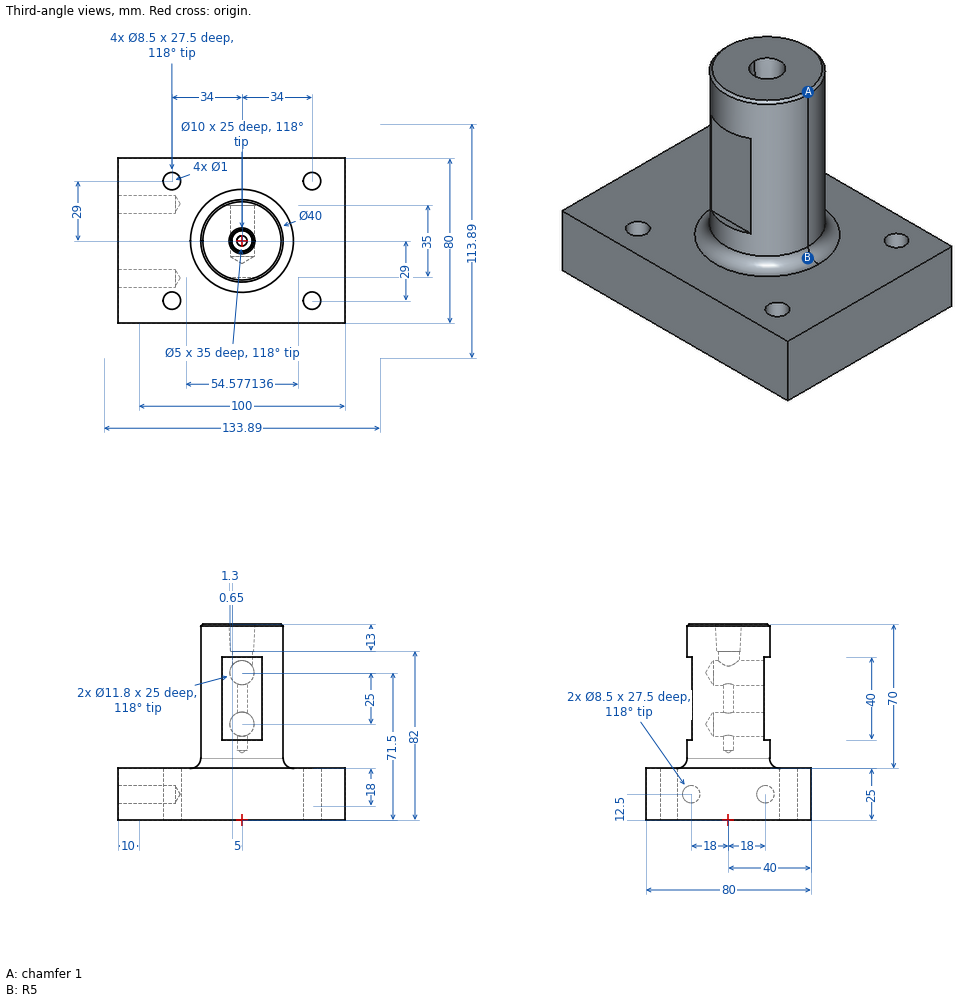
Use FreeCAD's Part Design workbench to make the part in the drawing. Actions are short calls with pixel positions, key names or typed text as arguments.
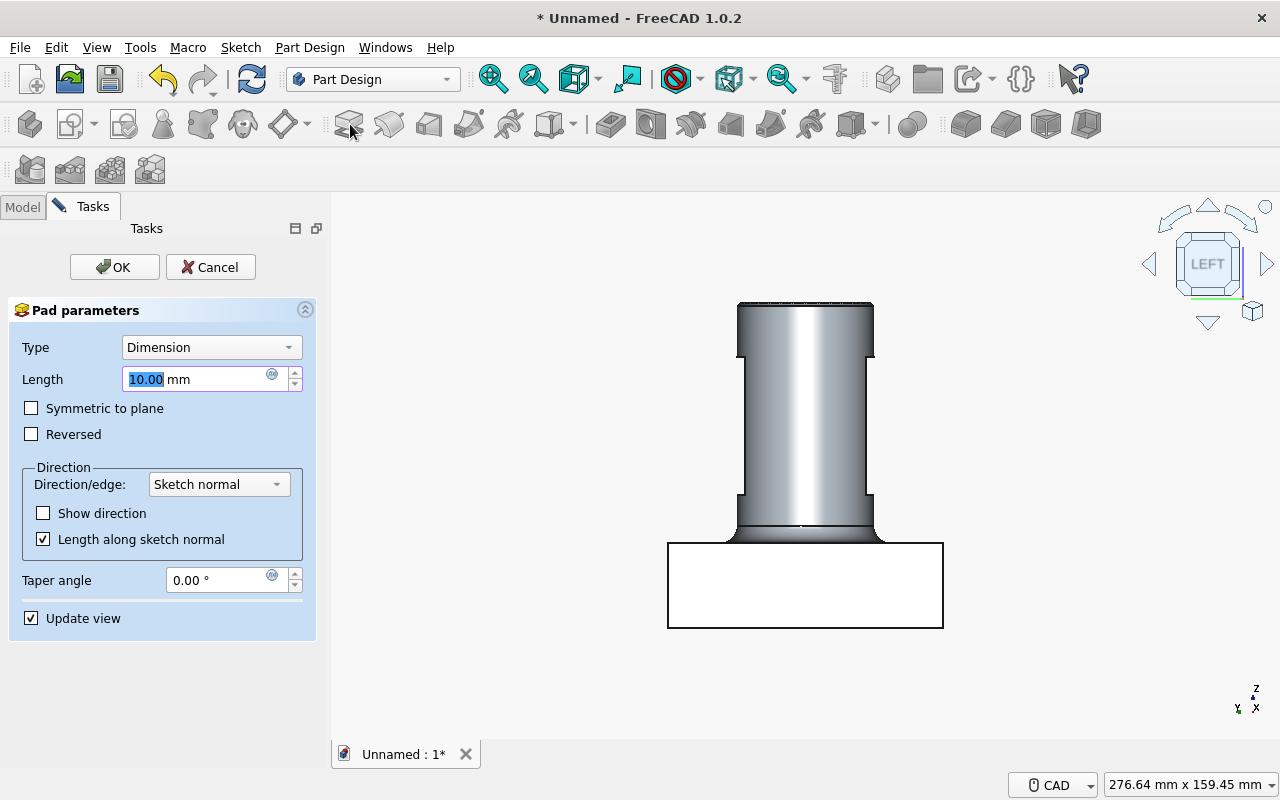
text(10)
key(Tab)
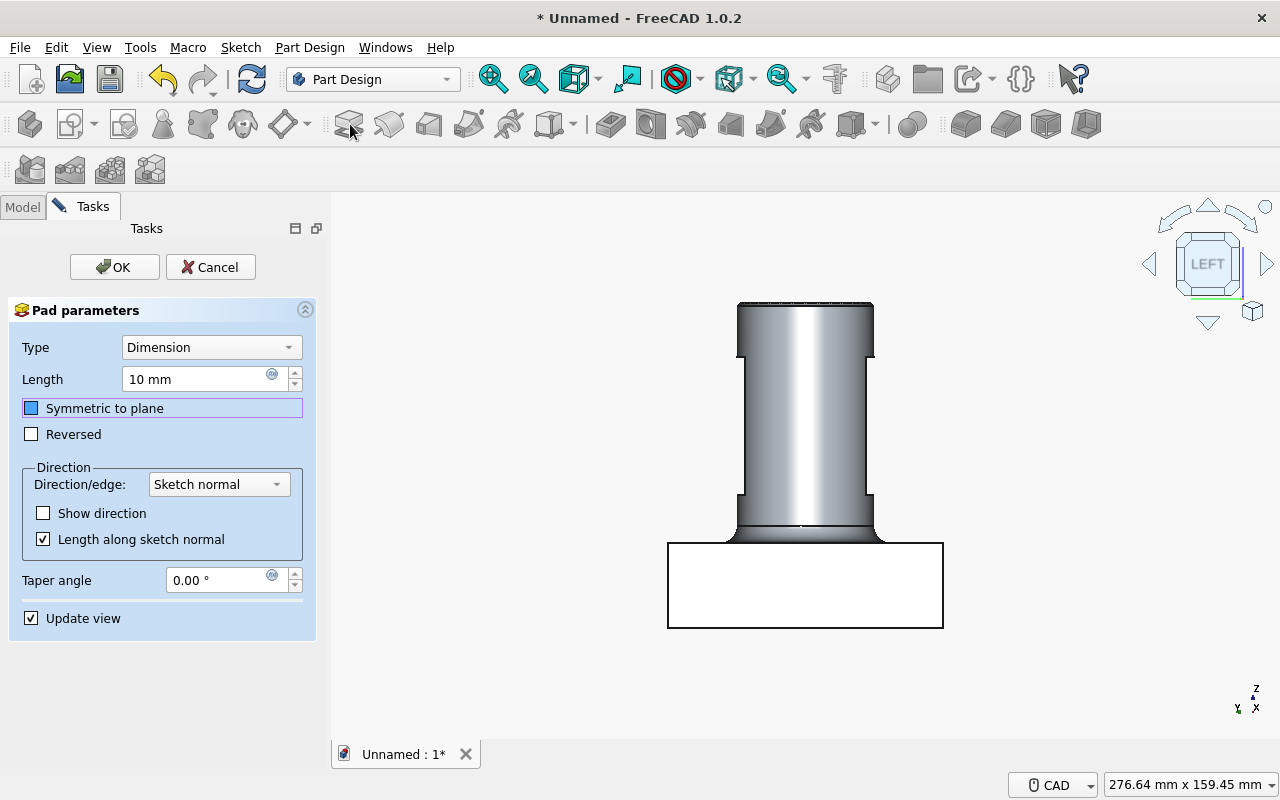
click(115, 267)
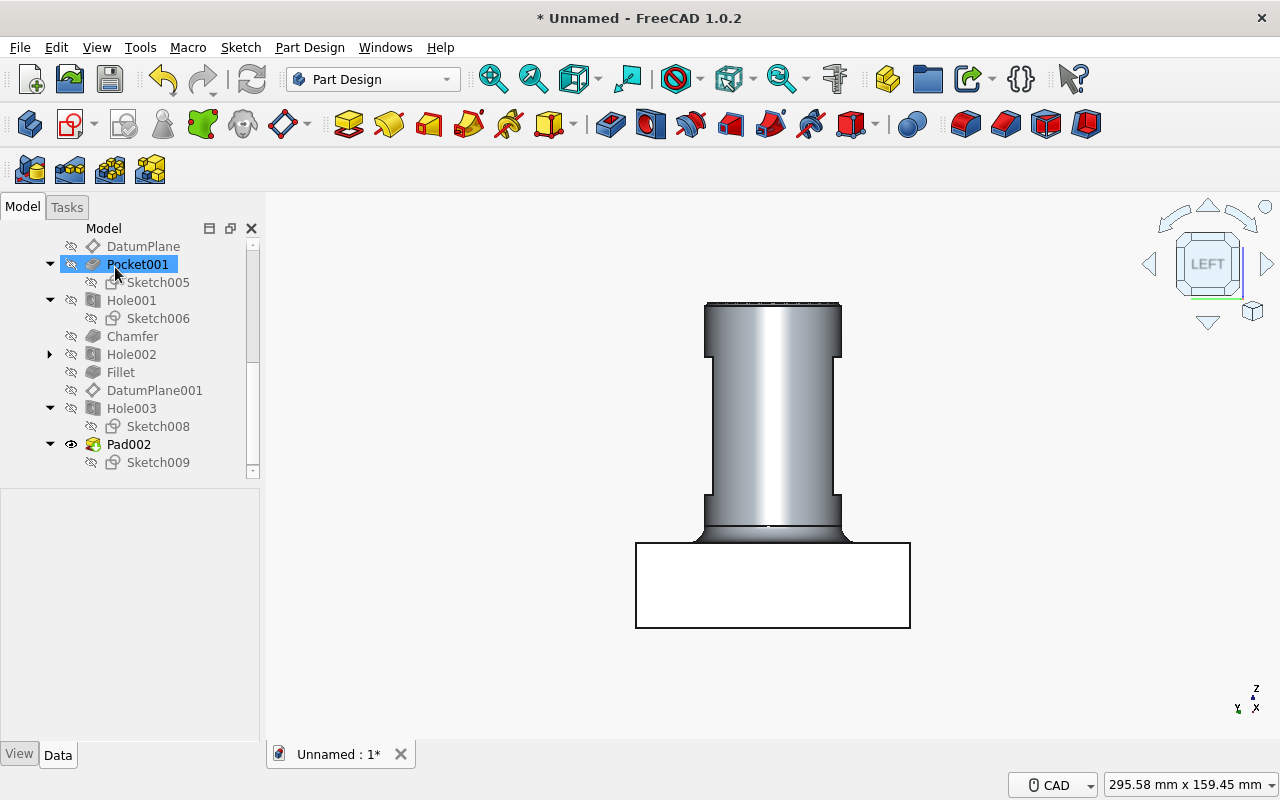
click(695, 585)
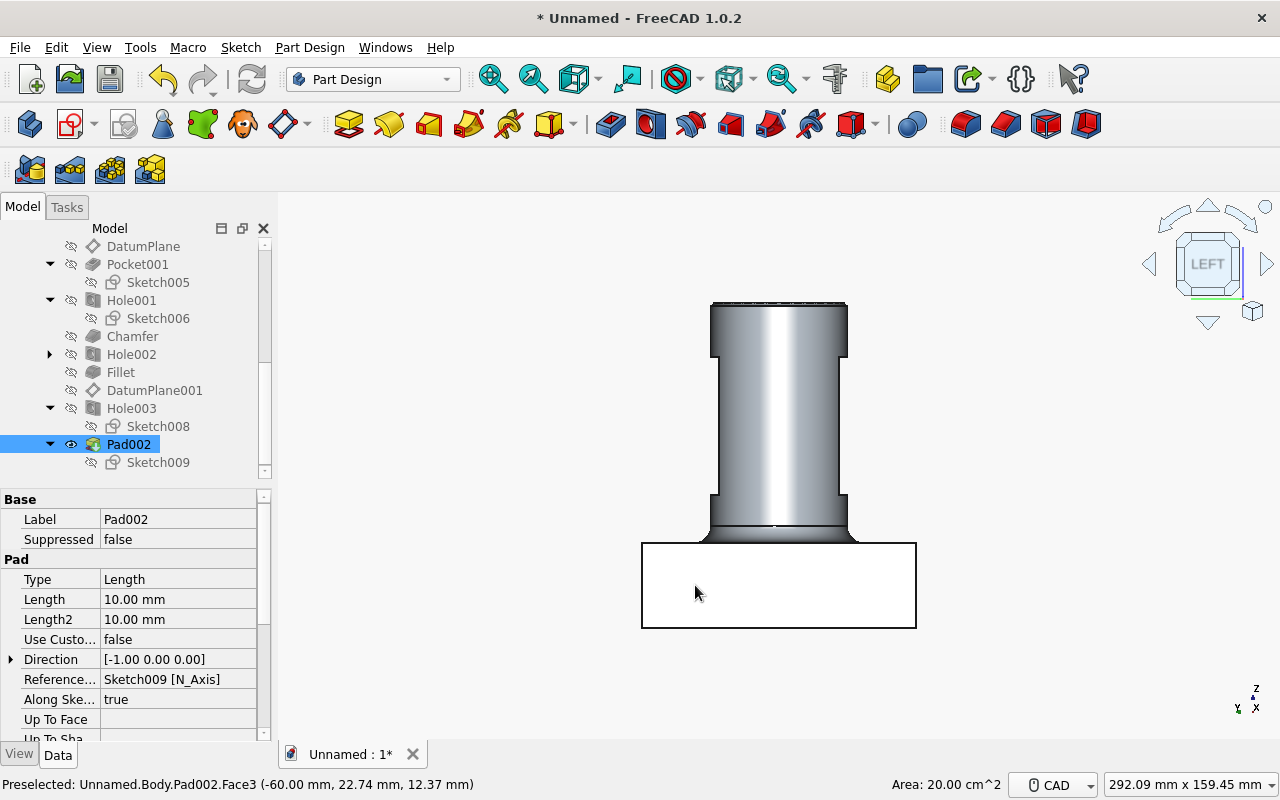
click(70, 124)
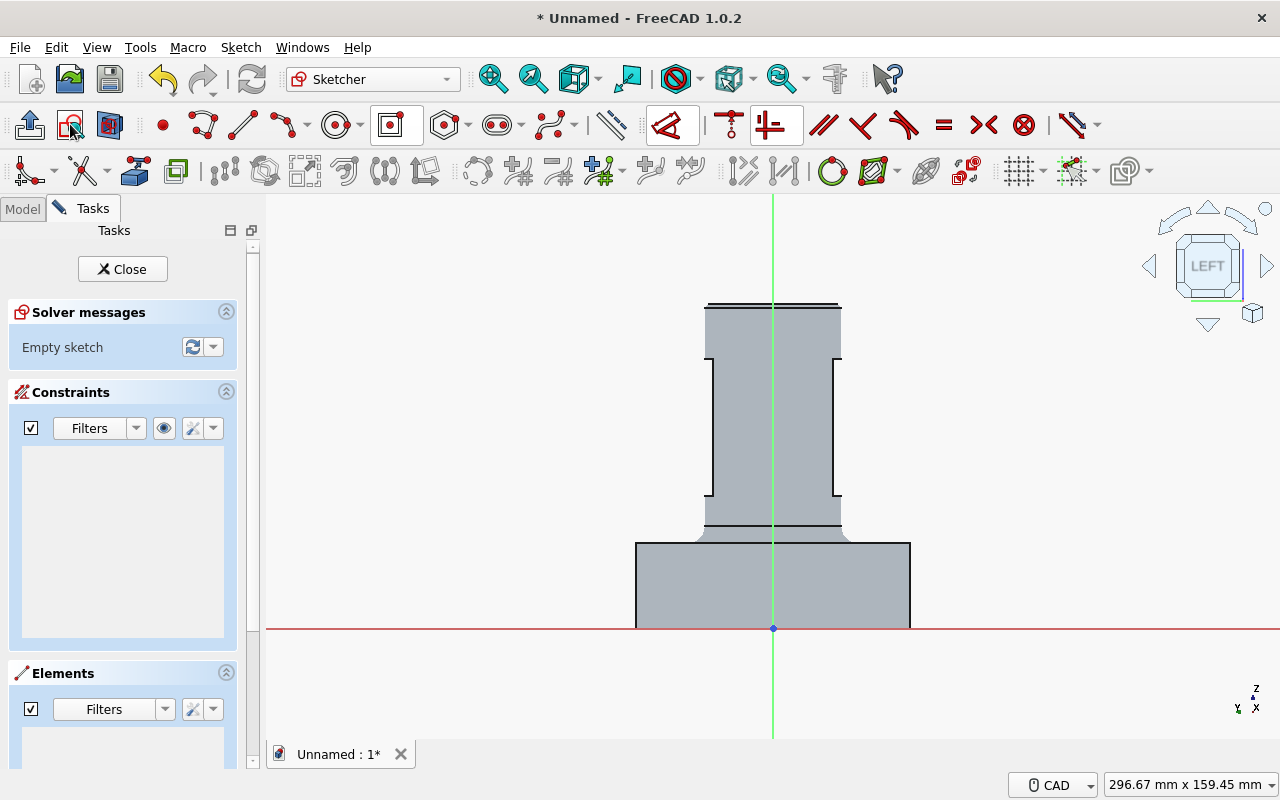
scroll(795, 644, up, 7)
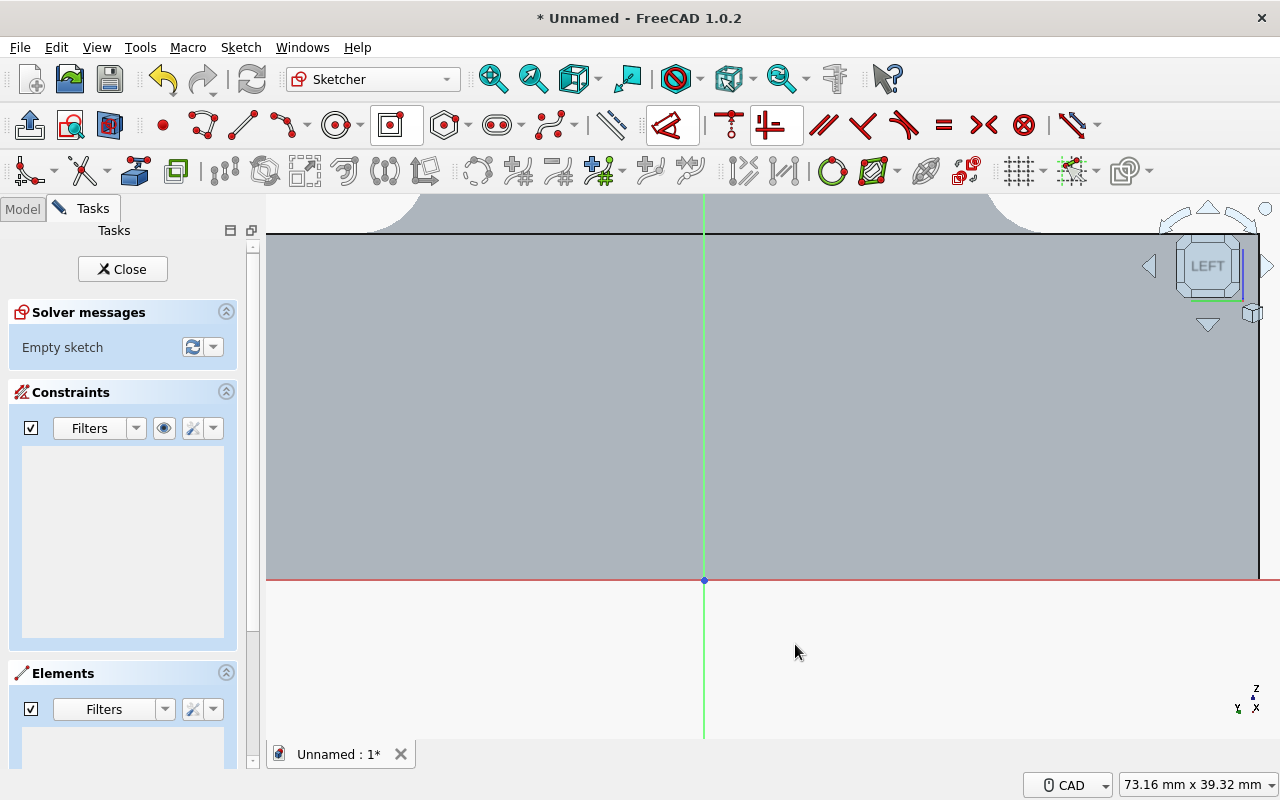
key(g)
key(c)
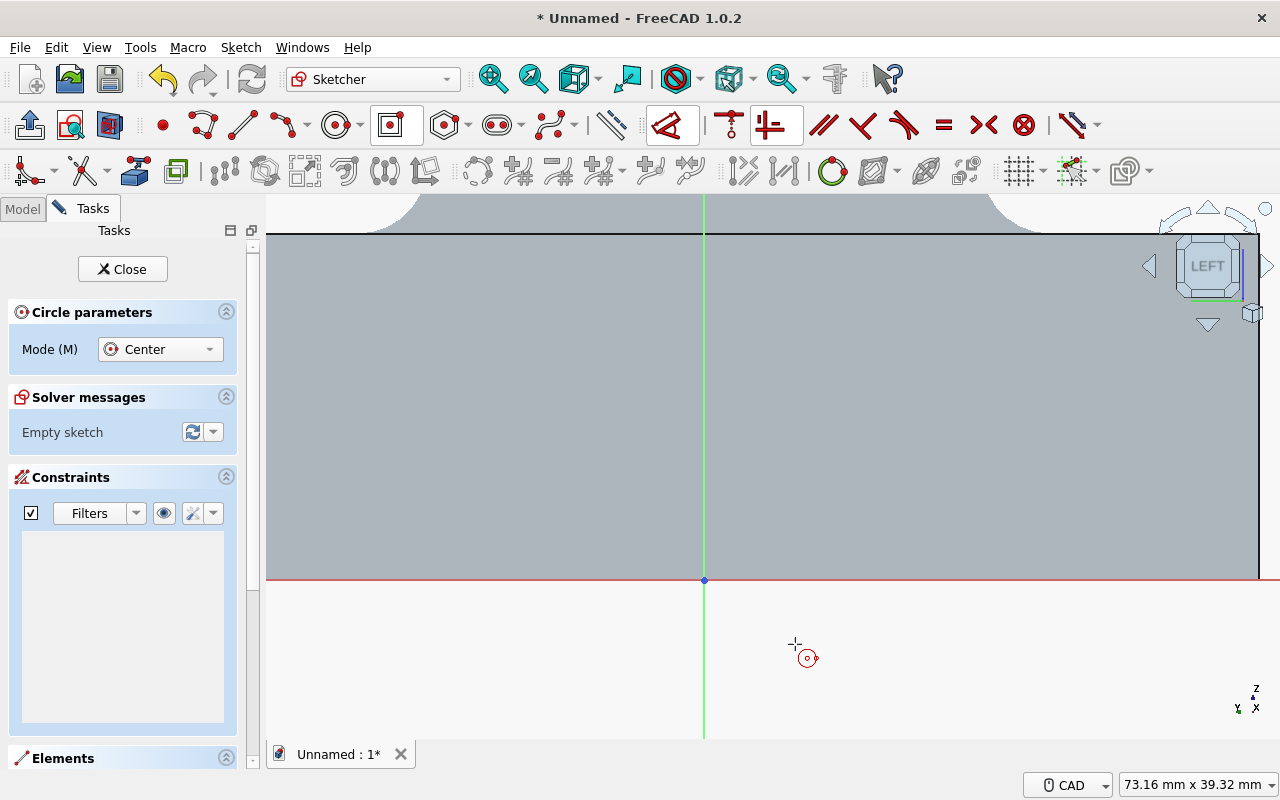
click(954, 407)
click(995, 365)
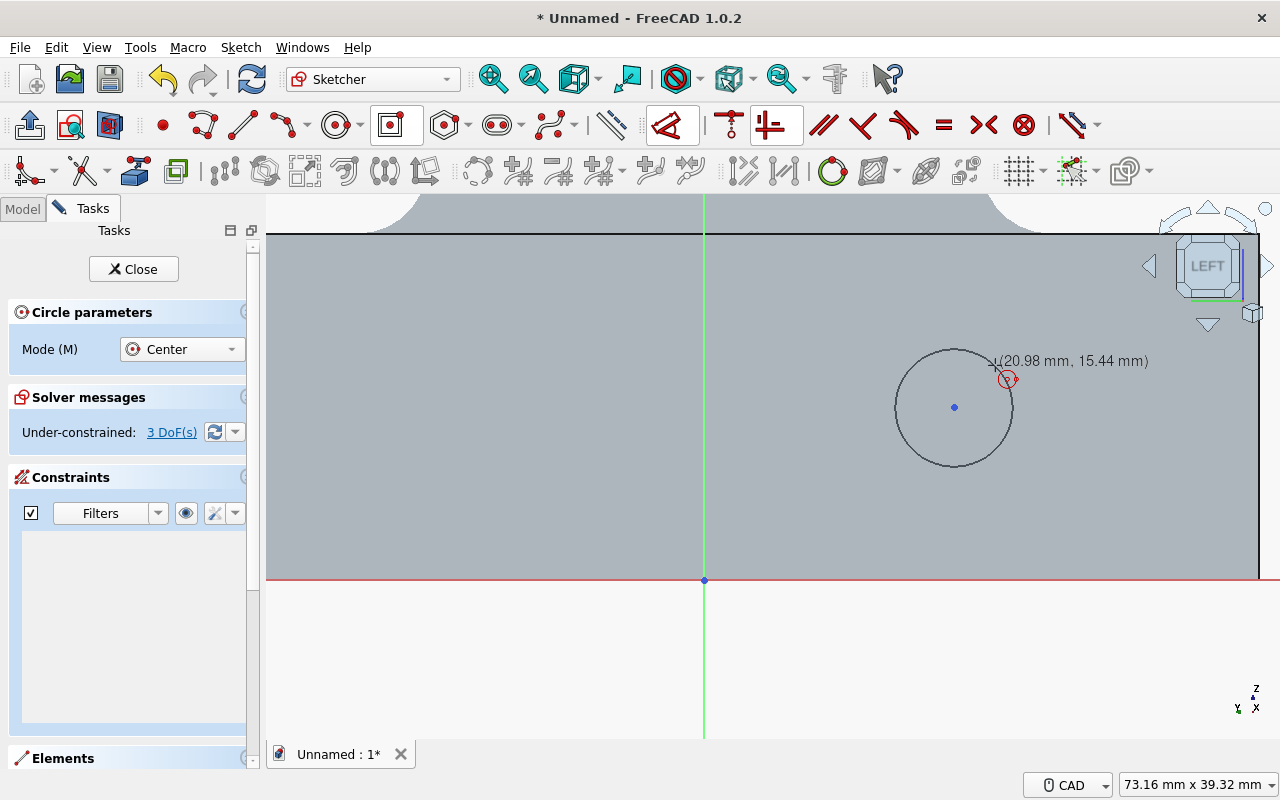
click(455, 407)
click(496, 365)
key(Escape)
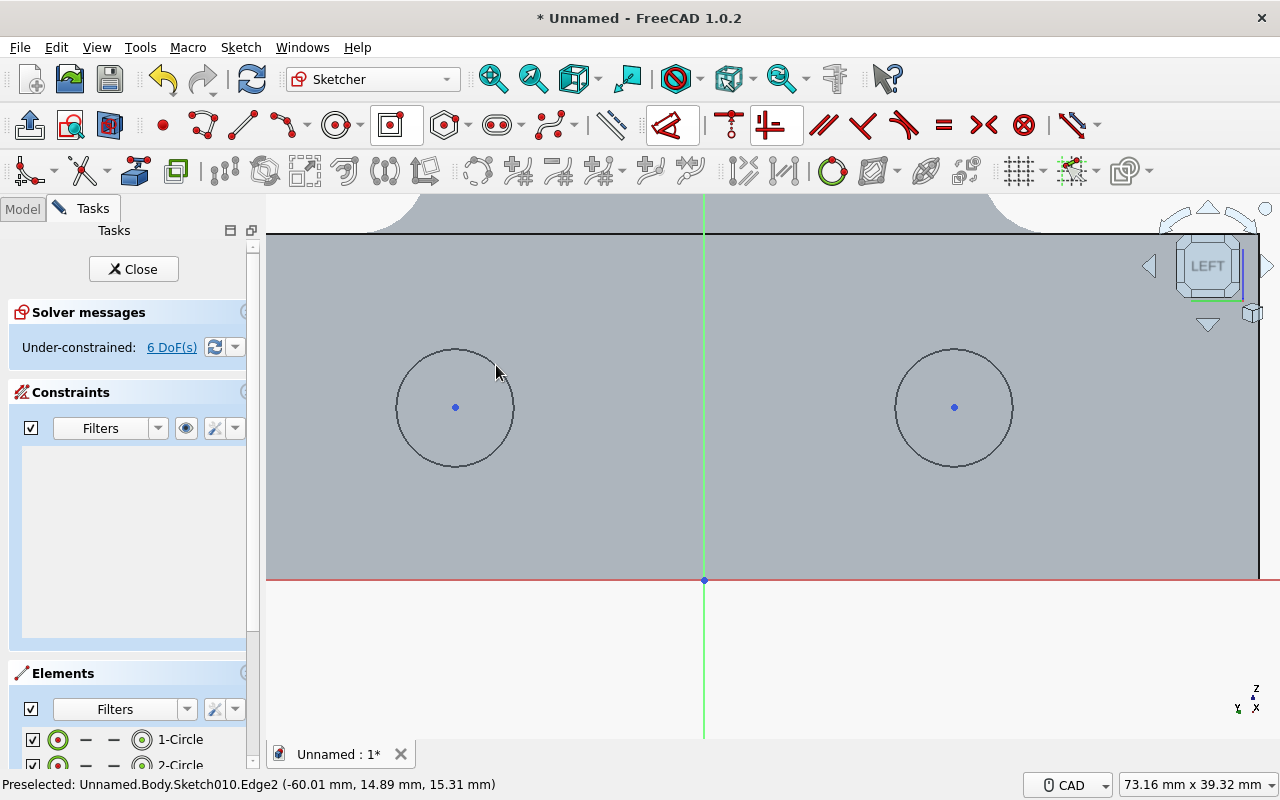
click(995, 366)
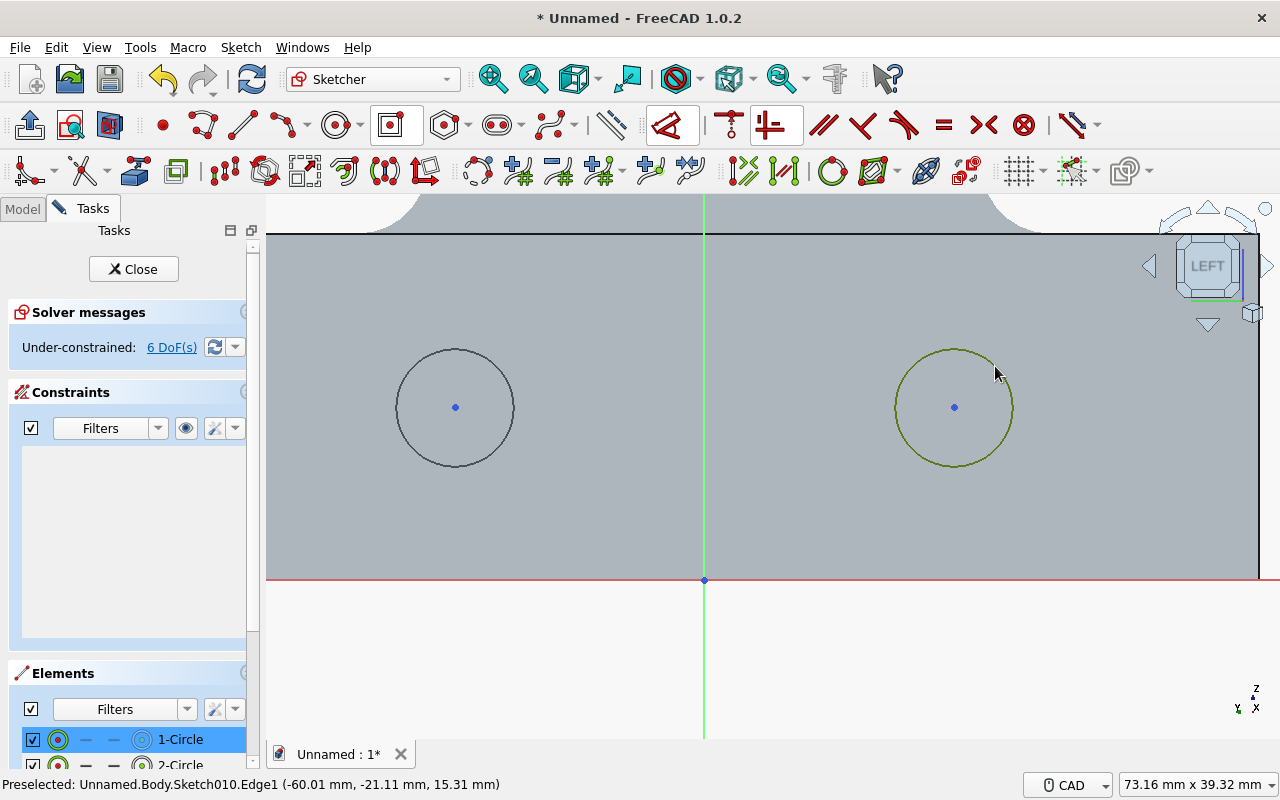
click(496, 366)